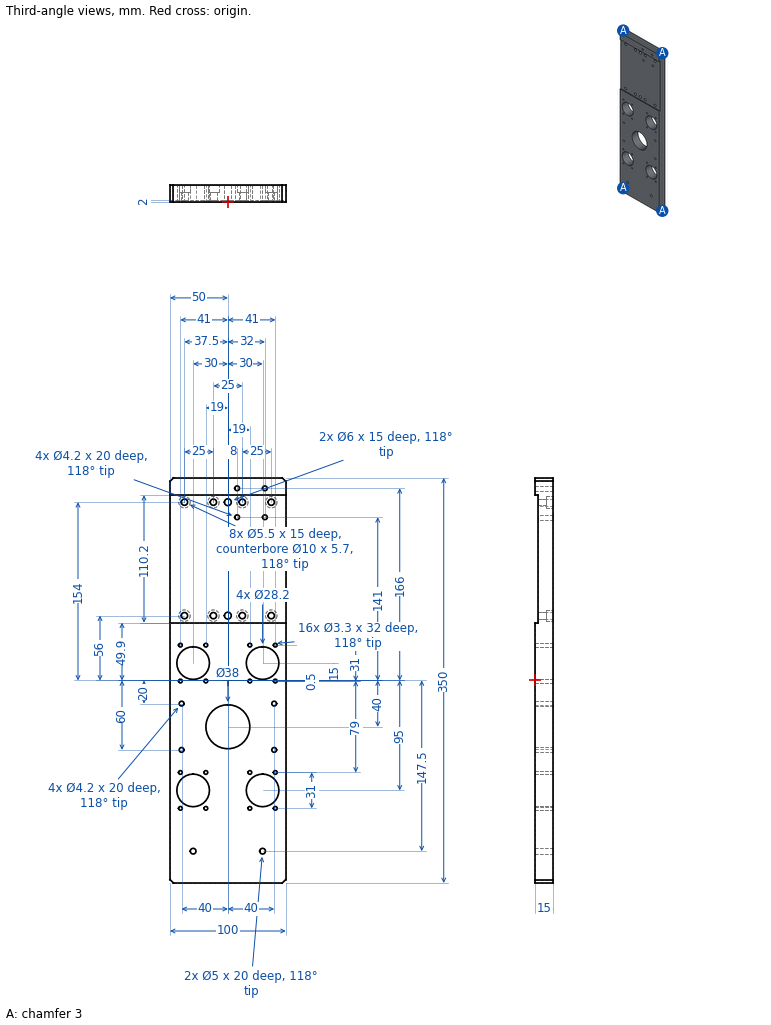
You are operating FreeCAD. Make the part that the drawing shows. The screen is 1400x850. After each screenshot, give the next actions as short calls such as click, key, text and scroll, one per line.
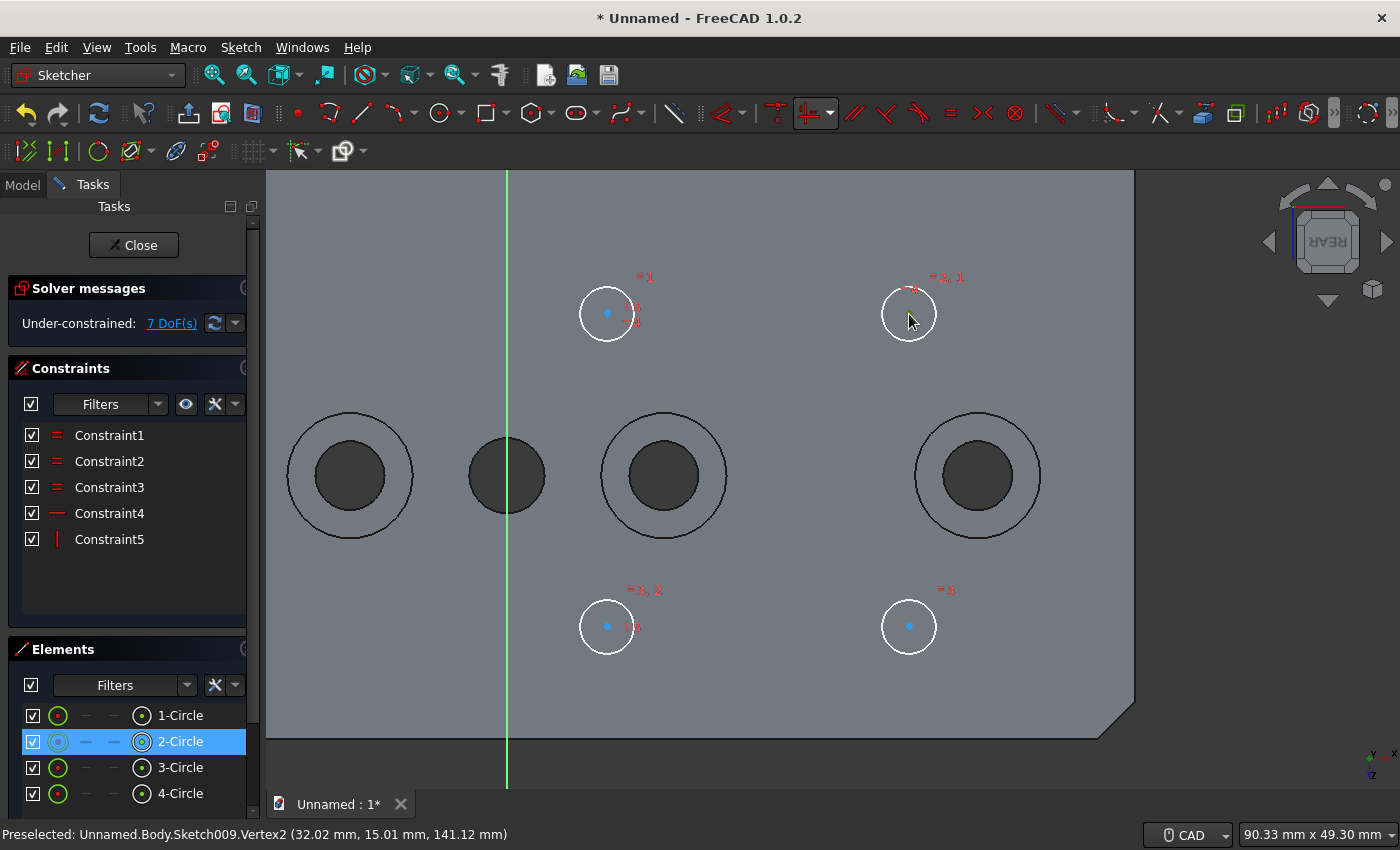
click(909, 627)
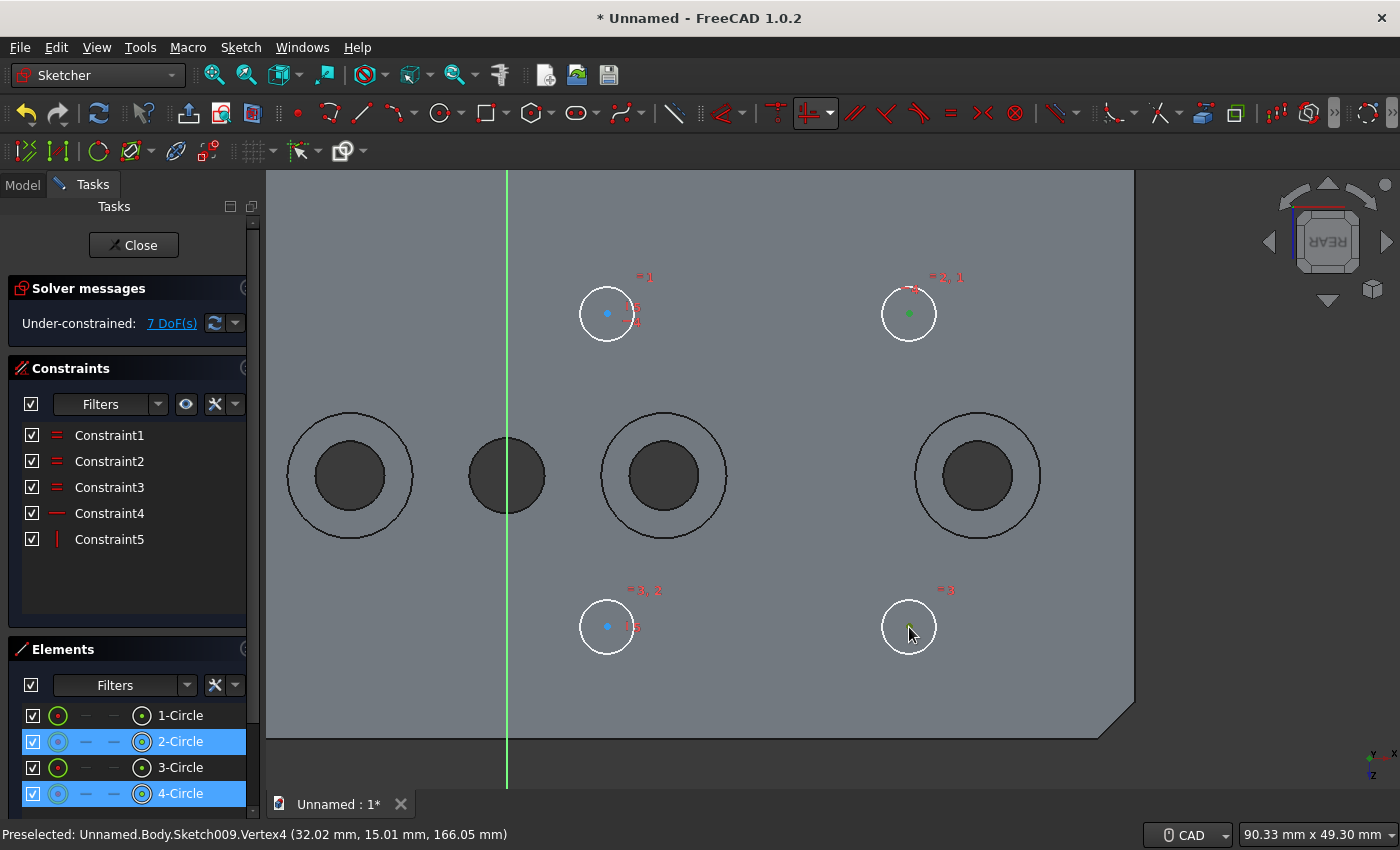
key(v)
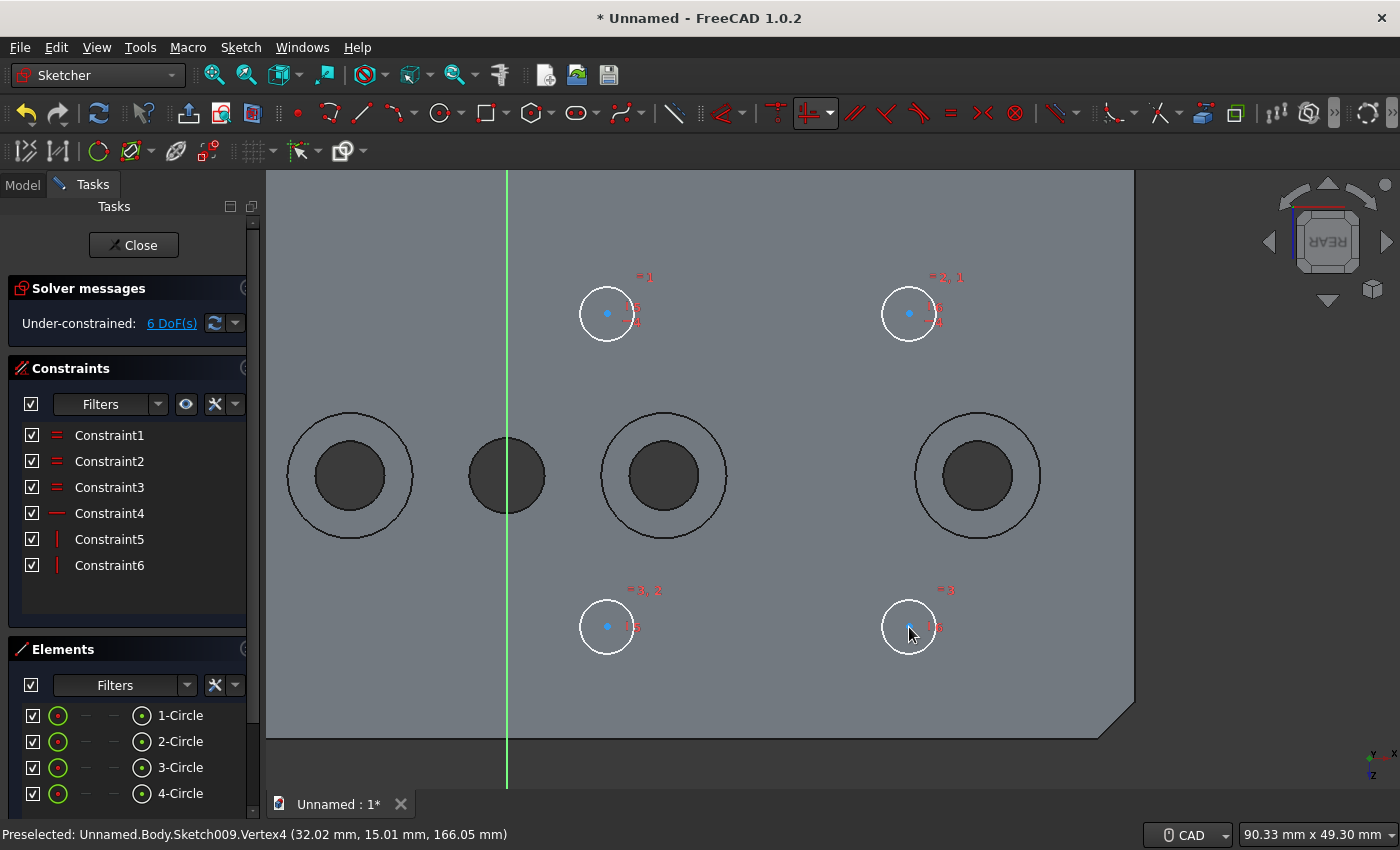
click(607, 627)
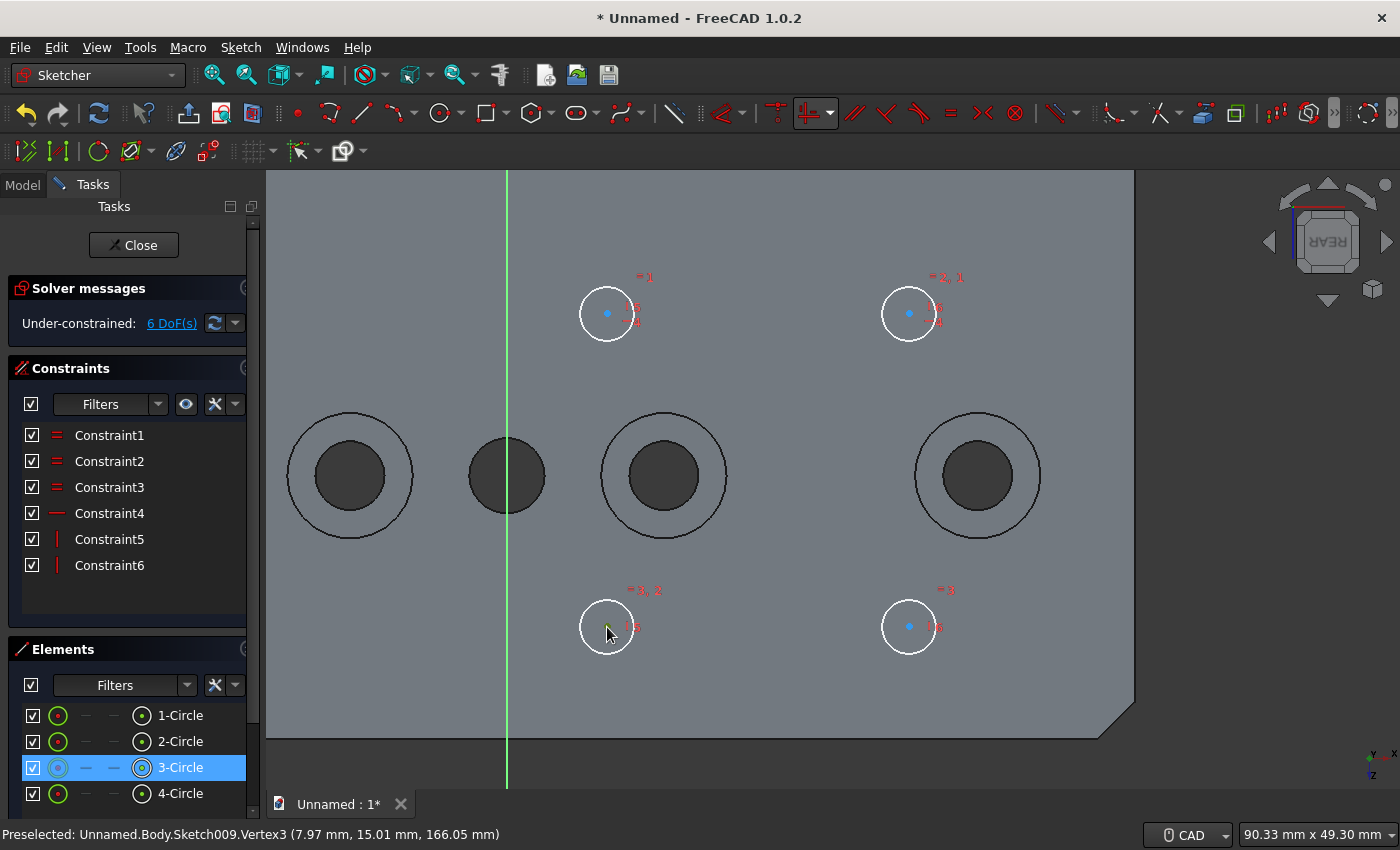
click(909, 627)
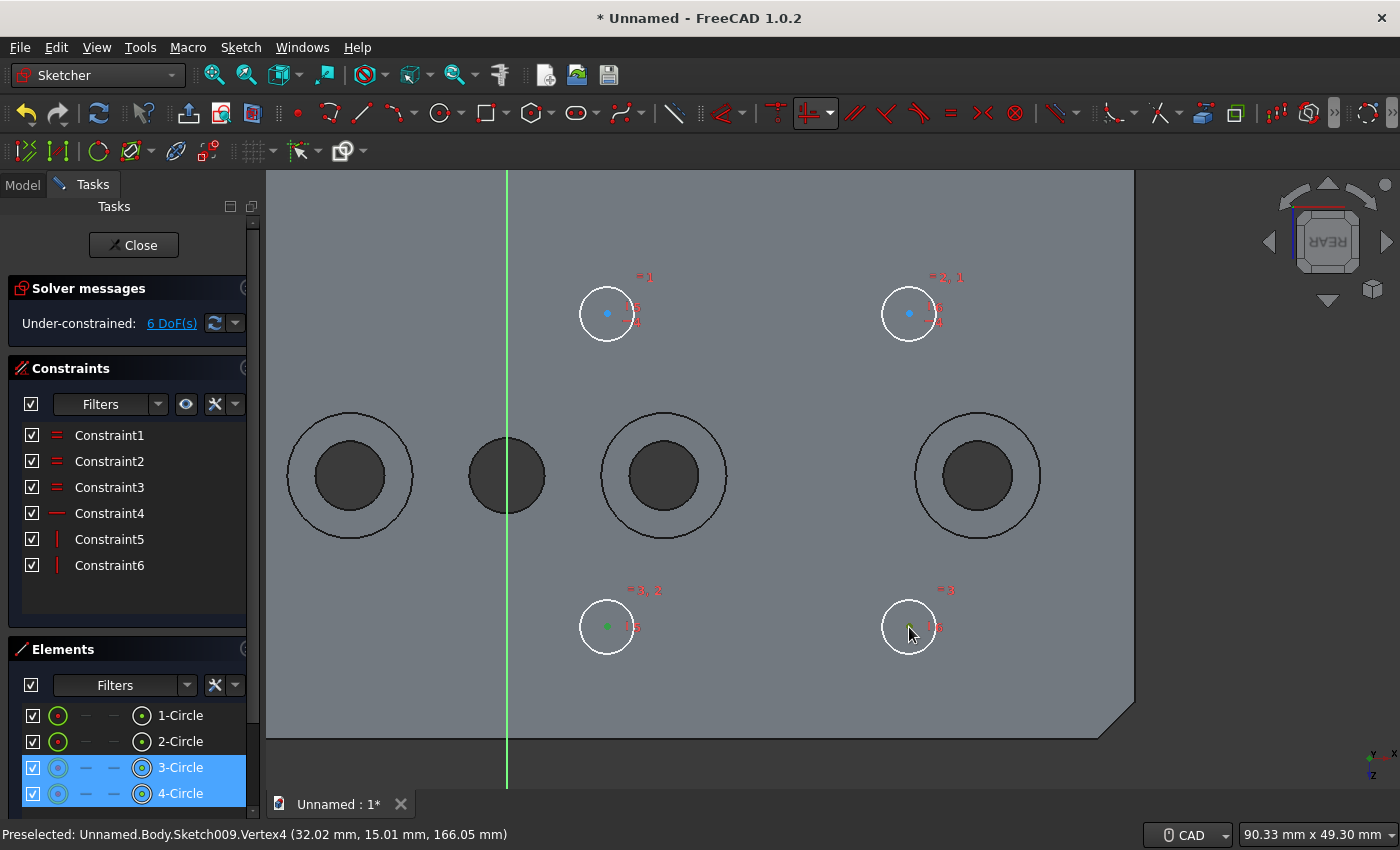
click(832, 114)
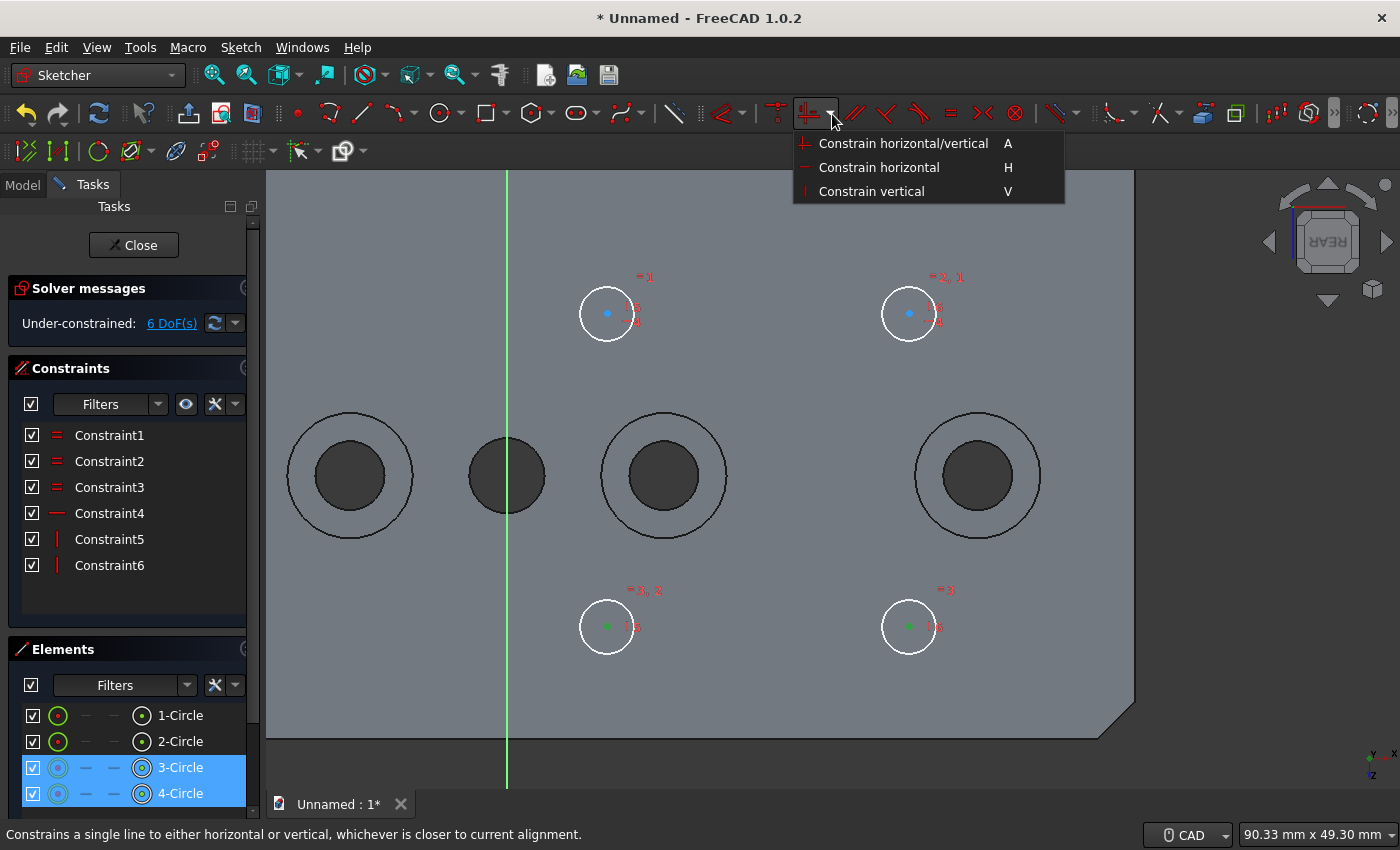
click(929, 167)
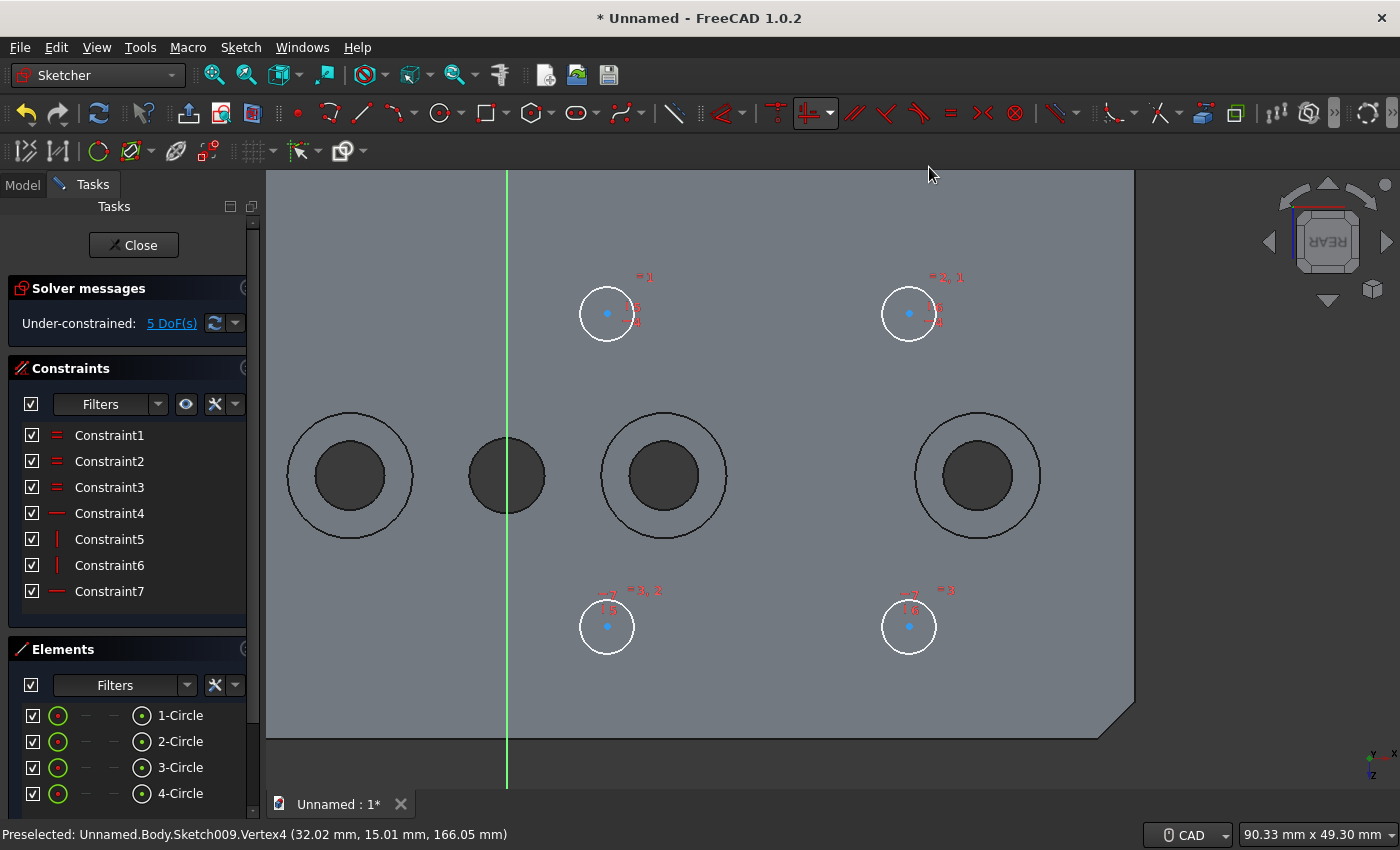
key(d)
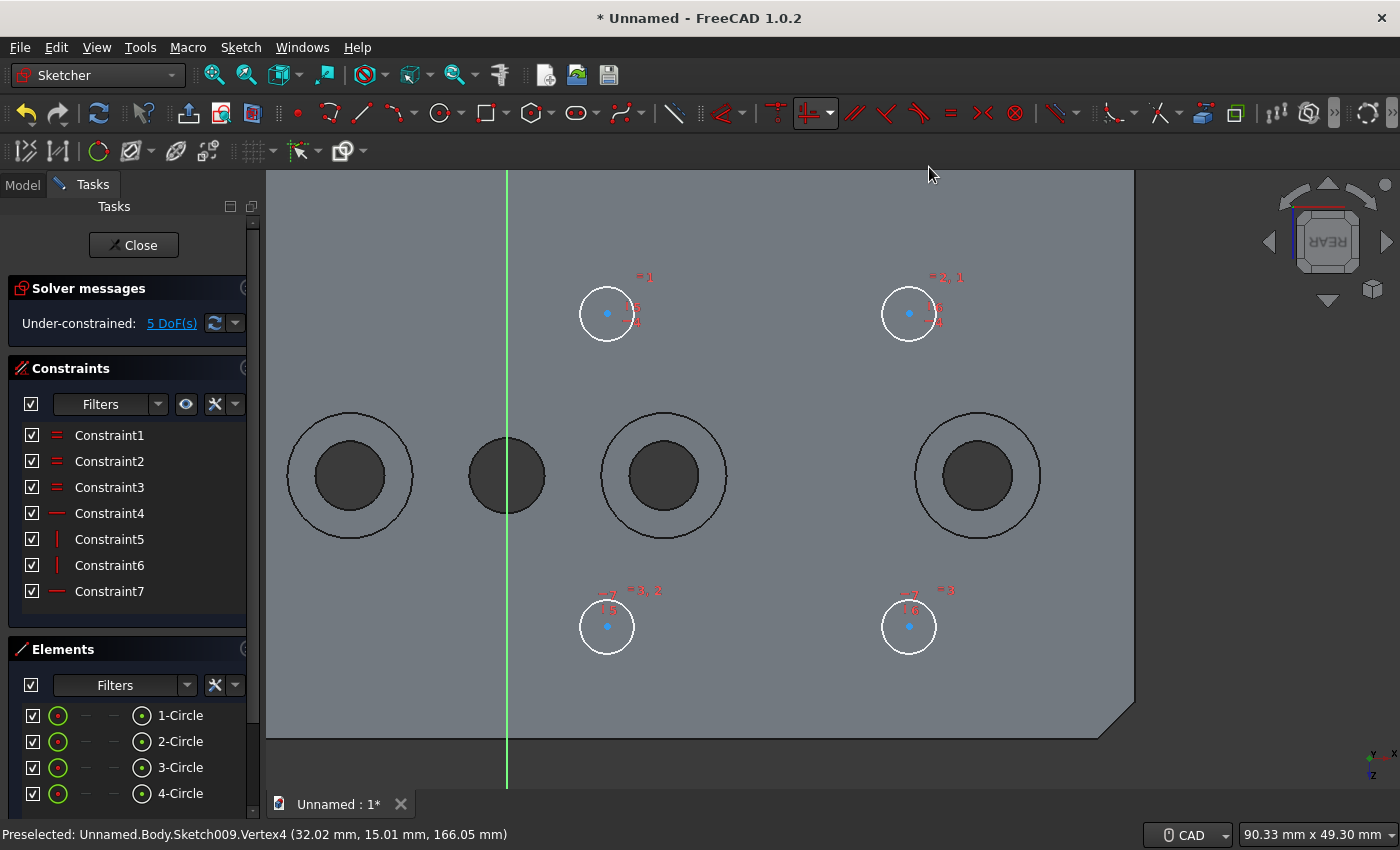
click(626, 295)
click(649, 272)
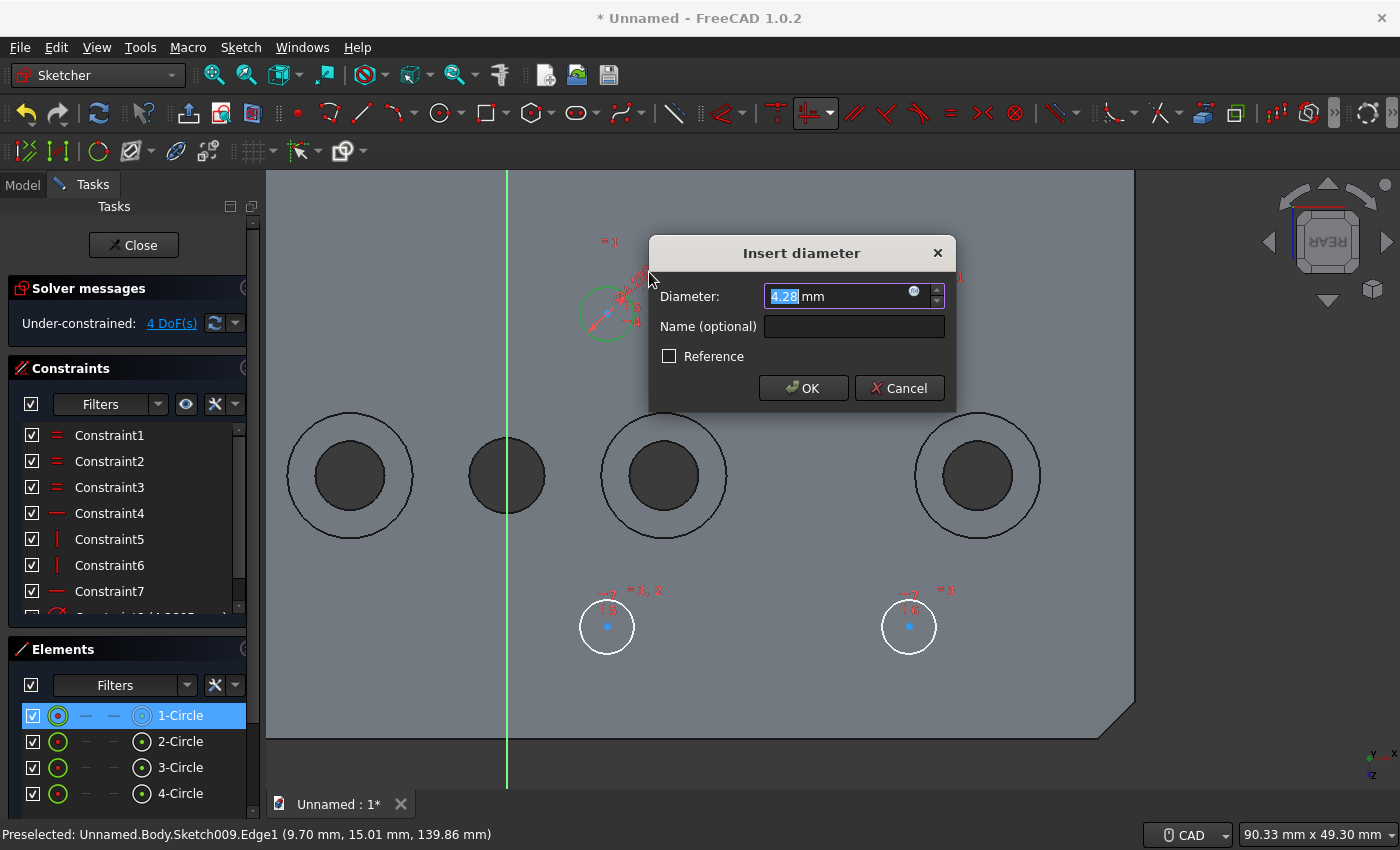
text(4.2)
key(Return)